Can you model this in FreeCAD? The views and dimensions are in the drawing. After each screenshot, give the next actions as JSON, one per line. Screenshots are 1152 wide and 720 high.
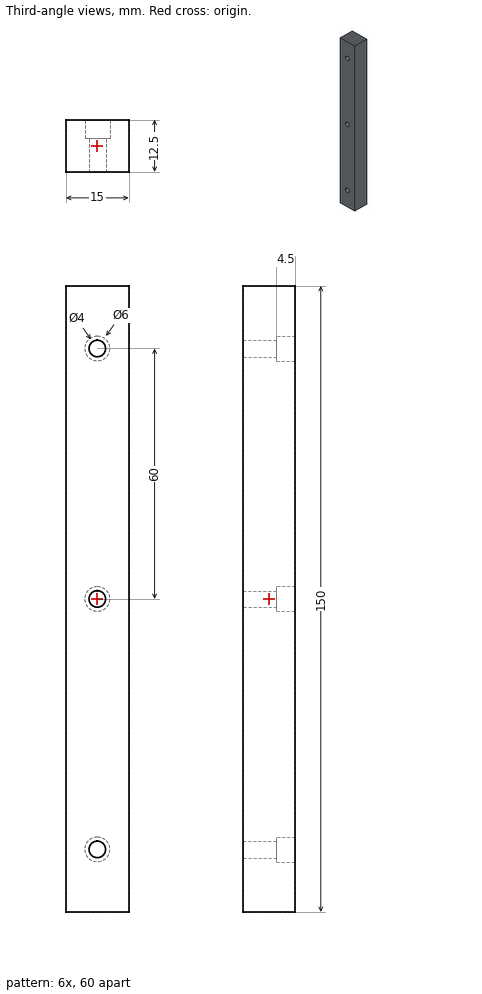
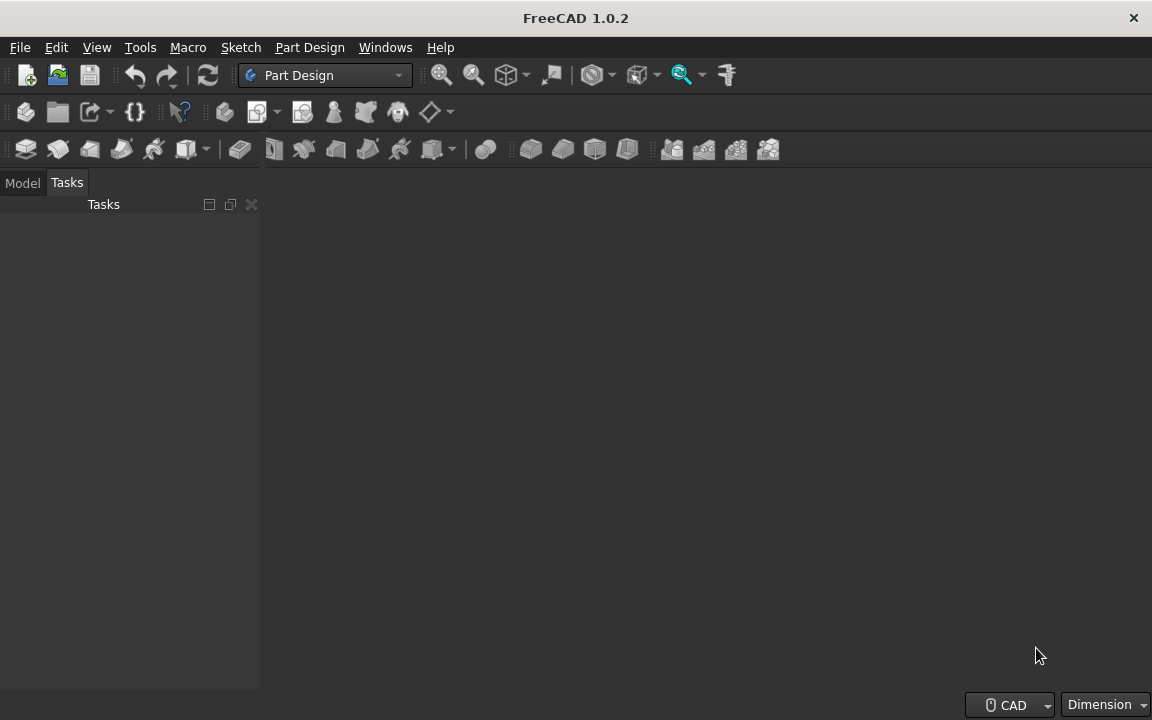
{"action": "key", "text": "ctrl+n"}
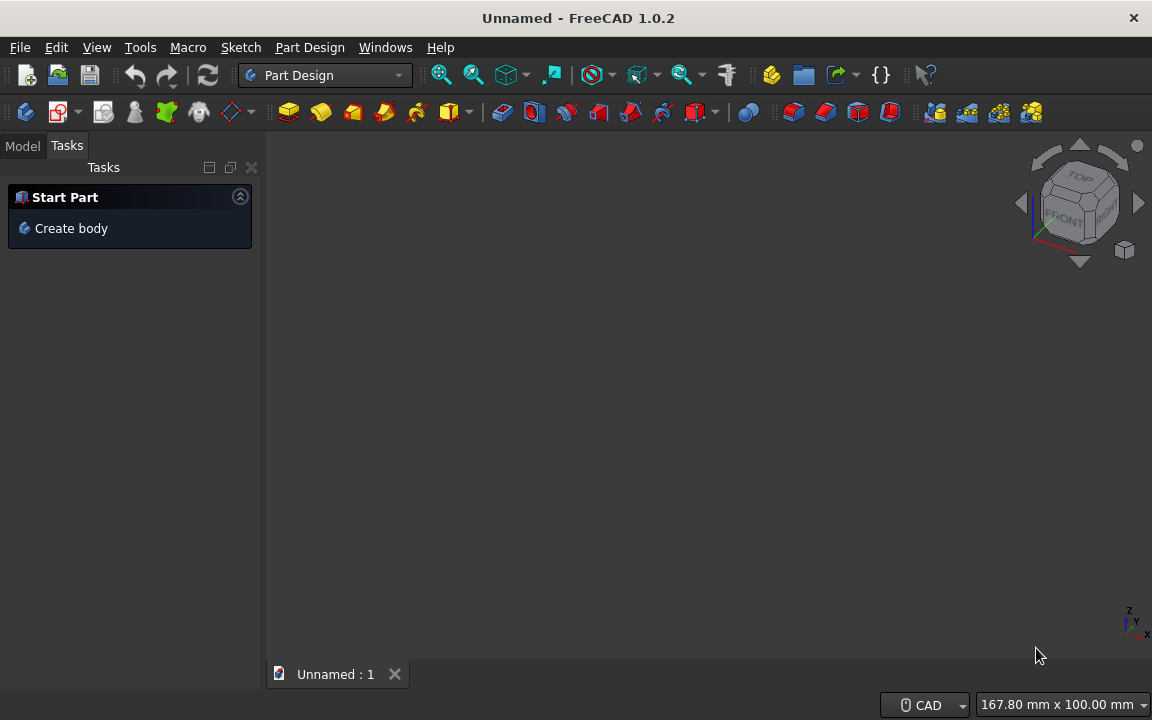
{"action": "left_click", "coordinate": [58, 112]}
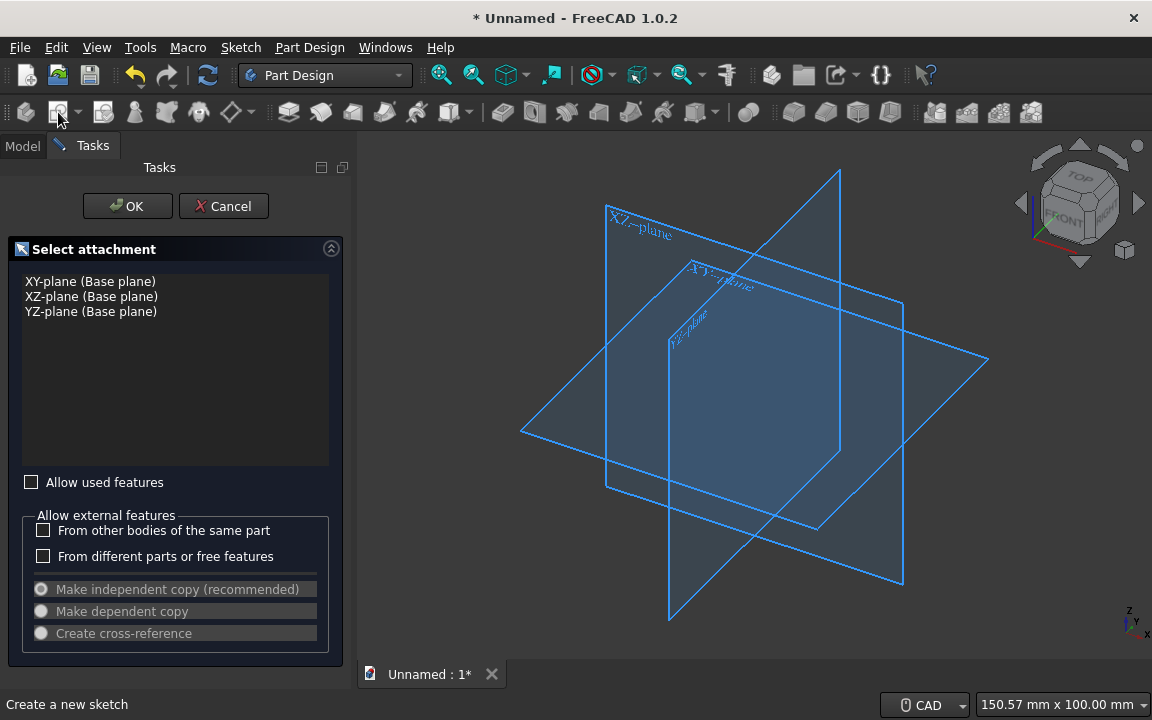
{"action": "left_click", "coordinate": [82, 282]}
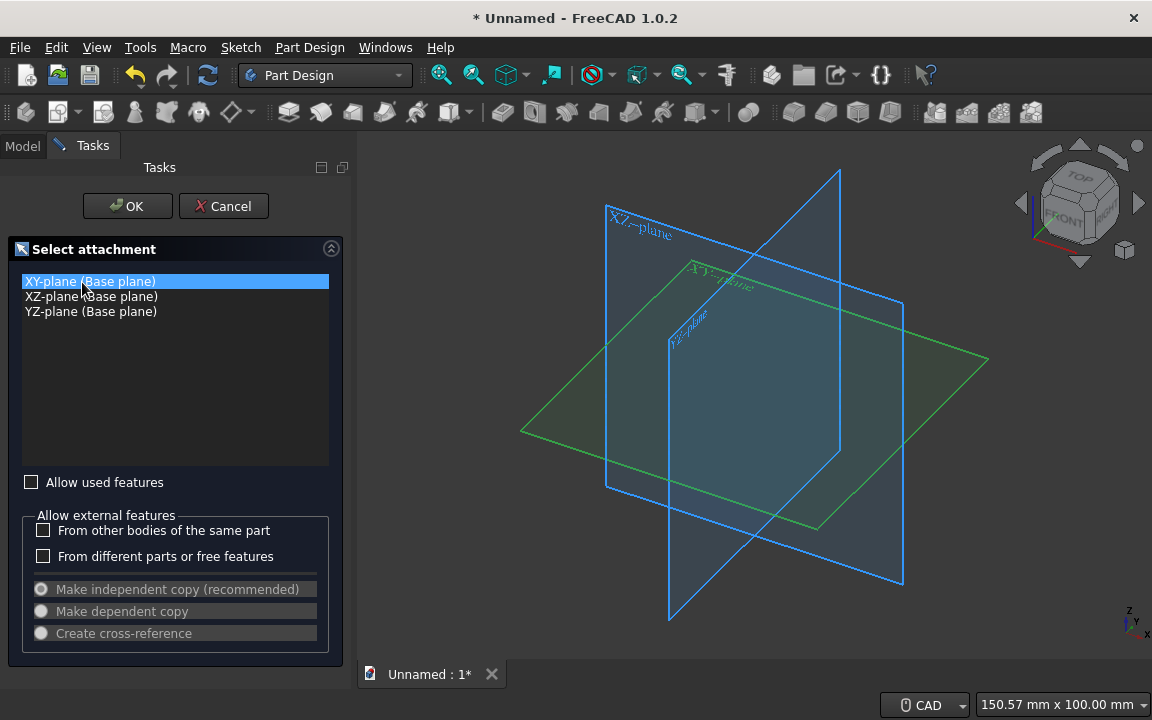
{"action": "left_click", "coordinate": [128, 206]}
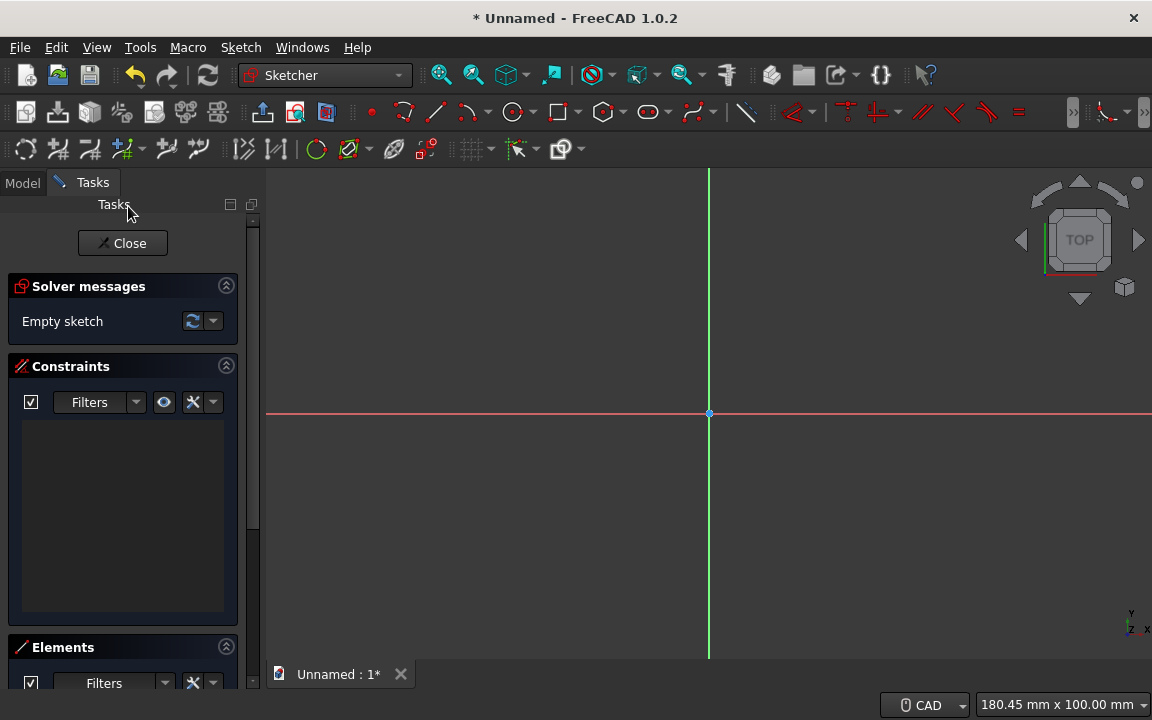
{"action": "scroll", "coordinate": [726, 414], "scroll_direction": "up", "scroll_amount": 8}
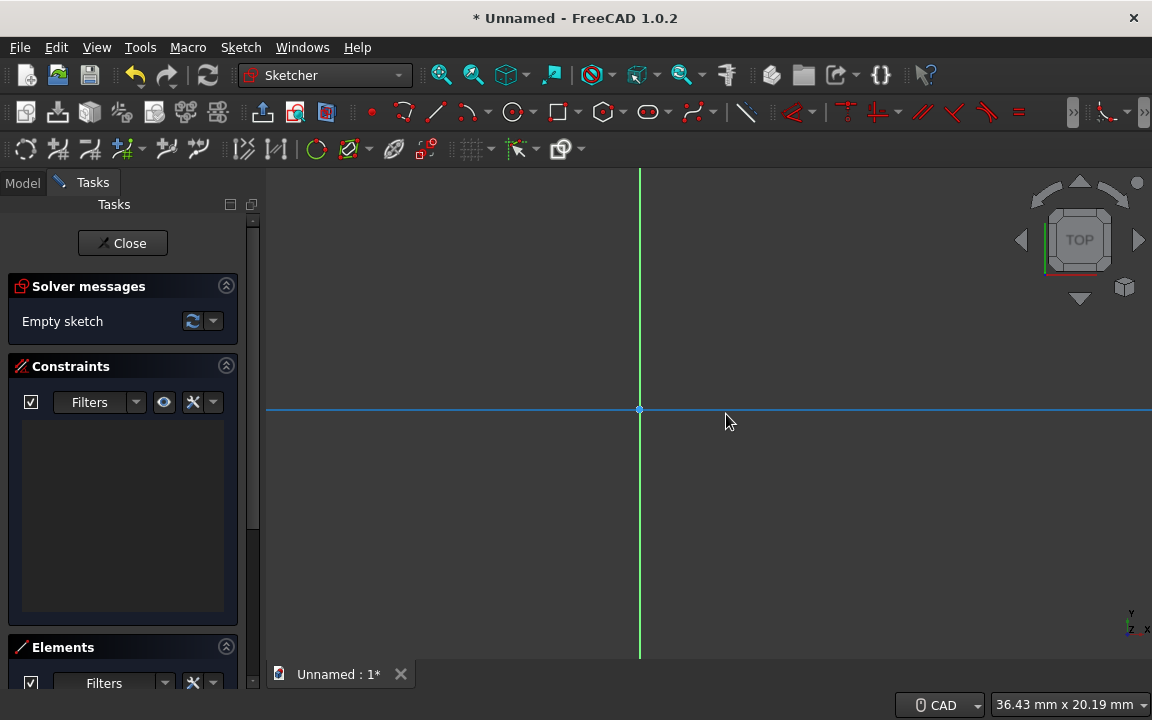
{"action": "key", "text": "g v"}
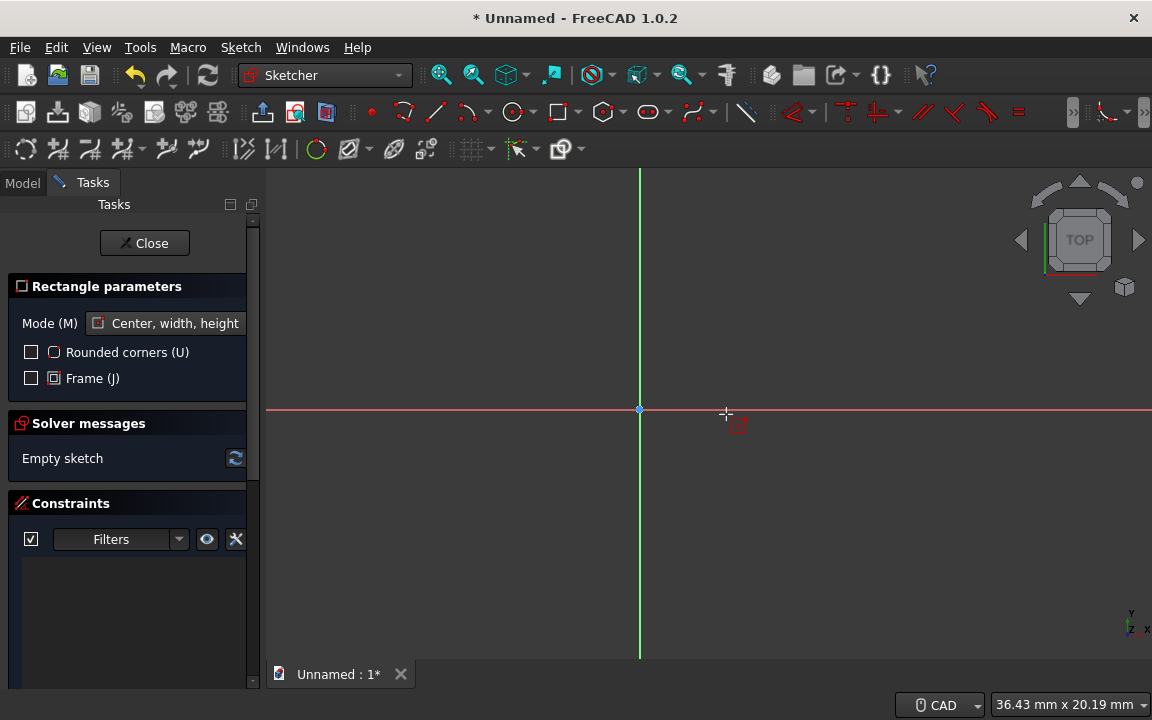
{"action": "left_click", "coordinate": [640, 410]}
{"action": "left_click", "coordinate": [822, 258]}
{"action": "key", "text": "Escape"}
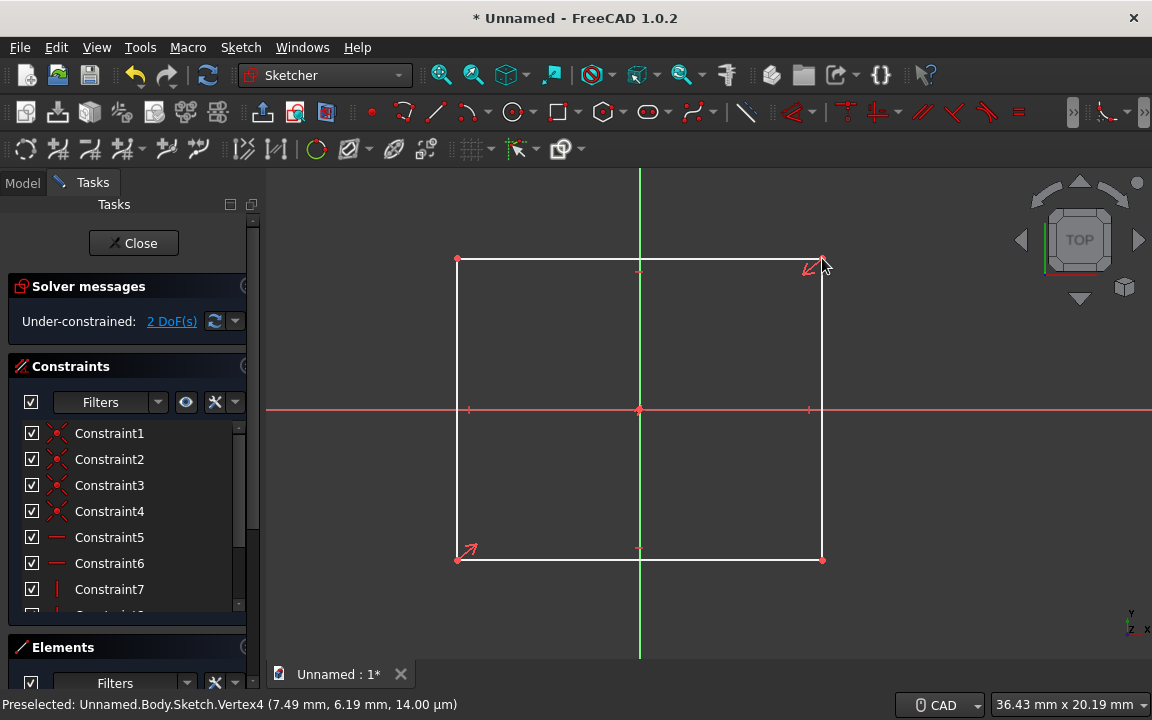
{"action": "left_click", "coordinate": [567, 560]}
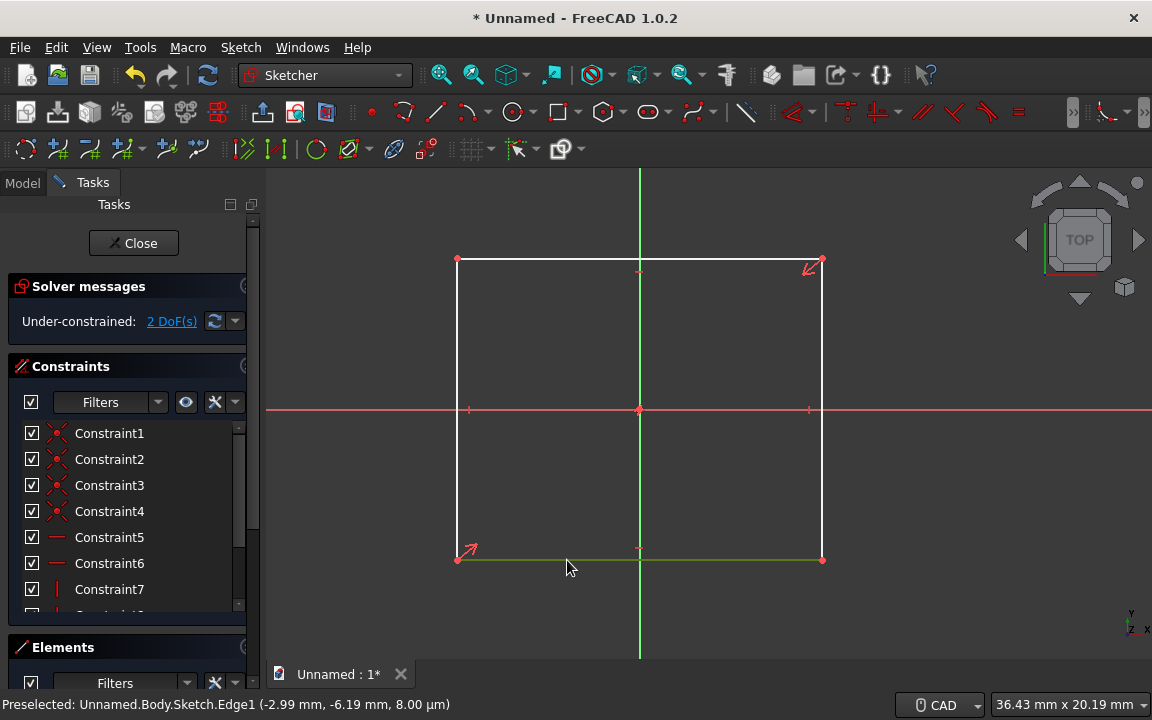
{"action": "left_click", "coordinate": [814, 112]}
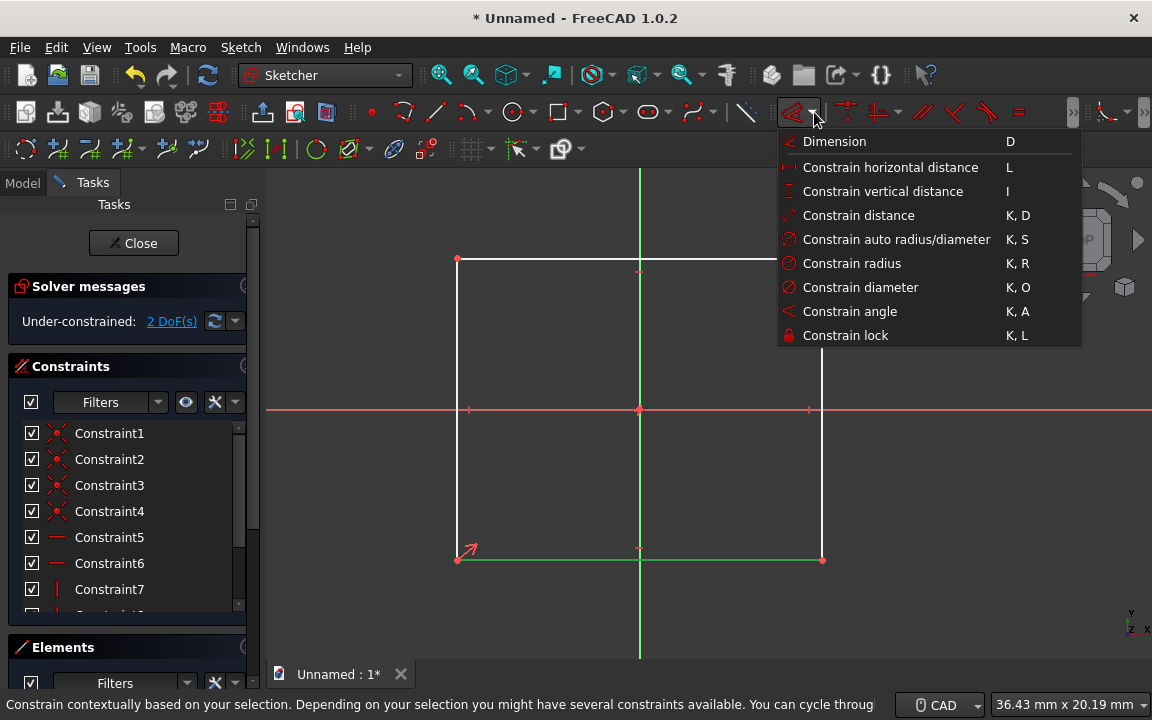
{"action": "left_click", "coordinate": [930, 167]}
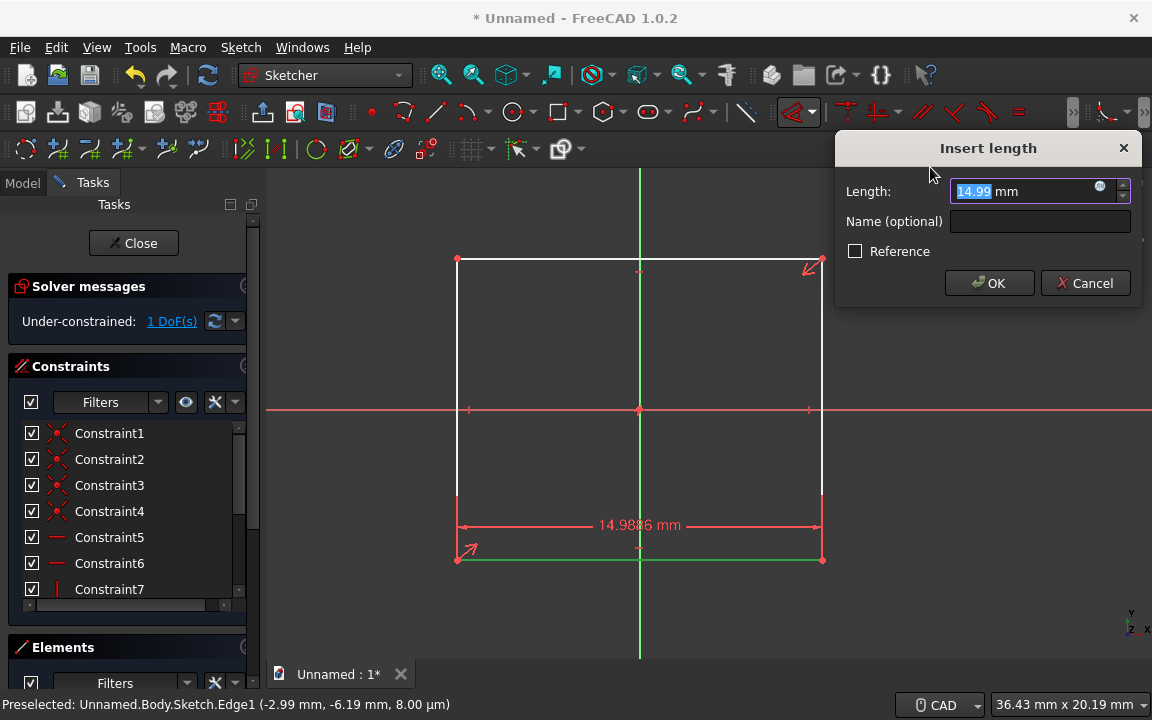
{"action": "type", "text": "15"}
{"action": "key", "text": "Return"}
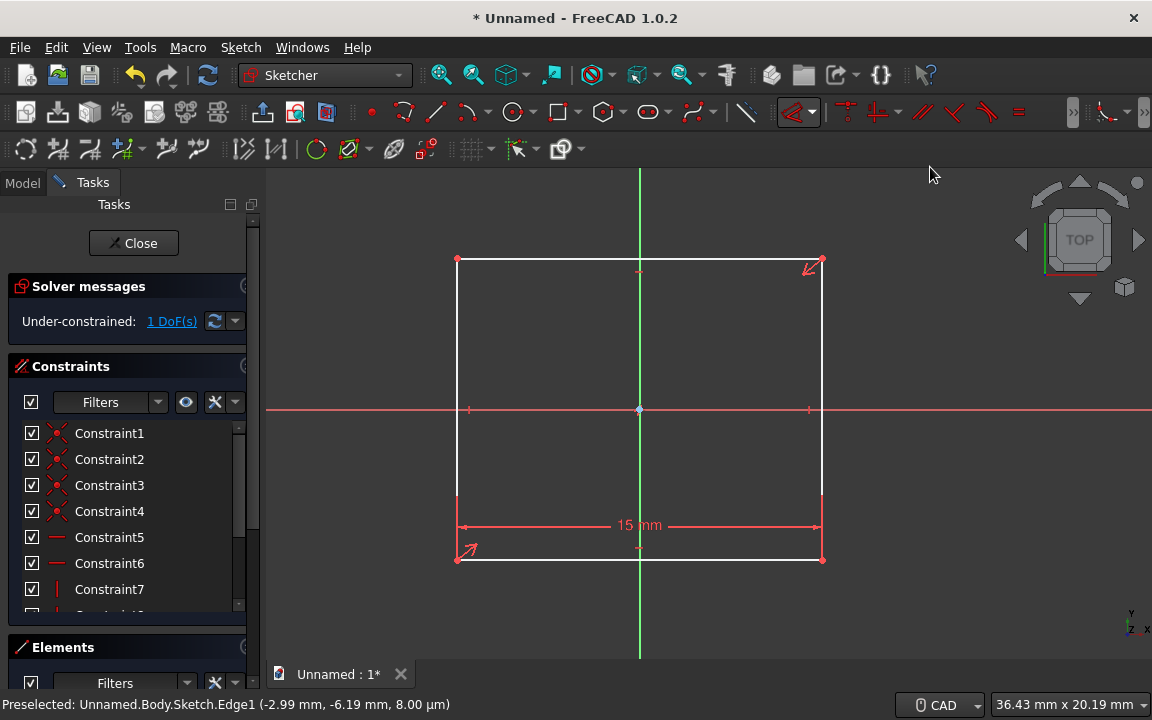
{"action": "left_click", "coordinate": [822, 470]}